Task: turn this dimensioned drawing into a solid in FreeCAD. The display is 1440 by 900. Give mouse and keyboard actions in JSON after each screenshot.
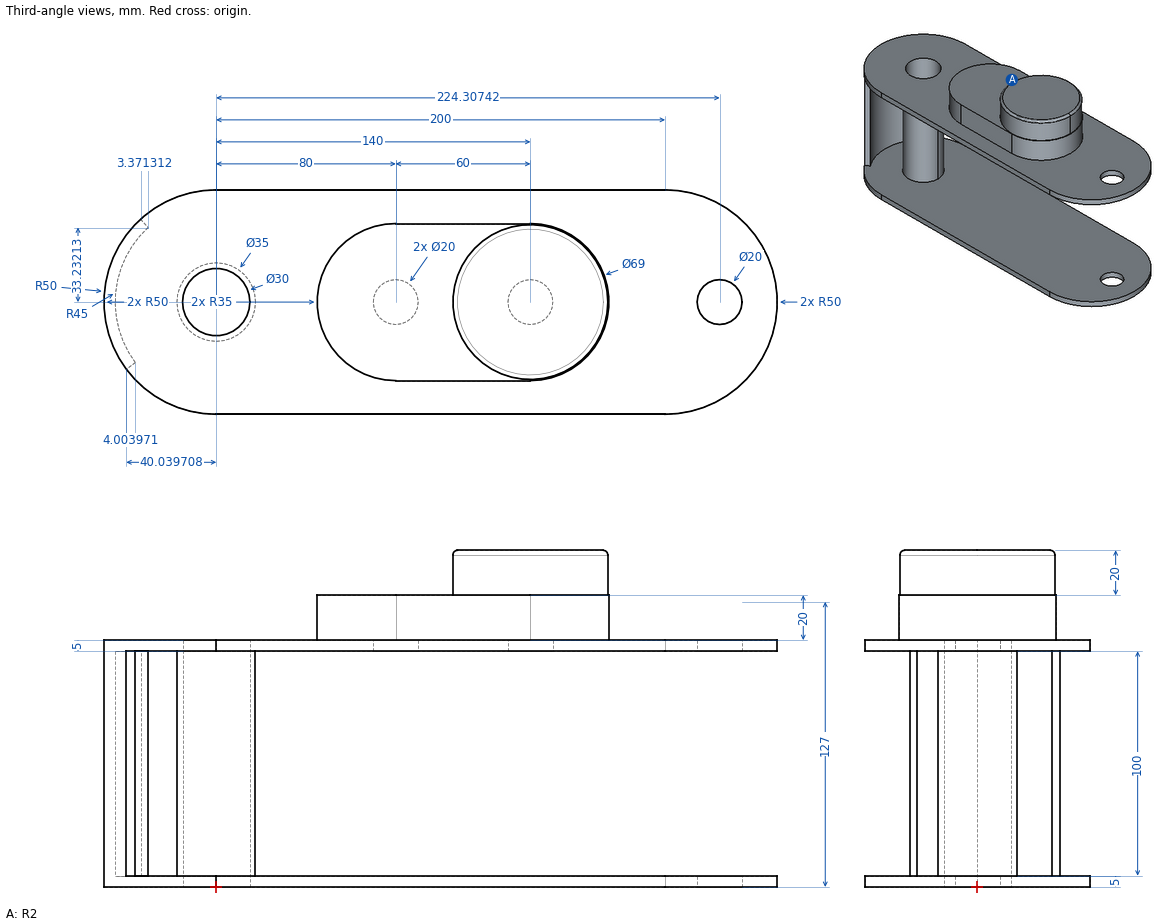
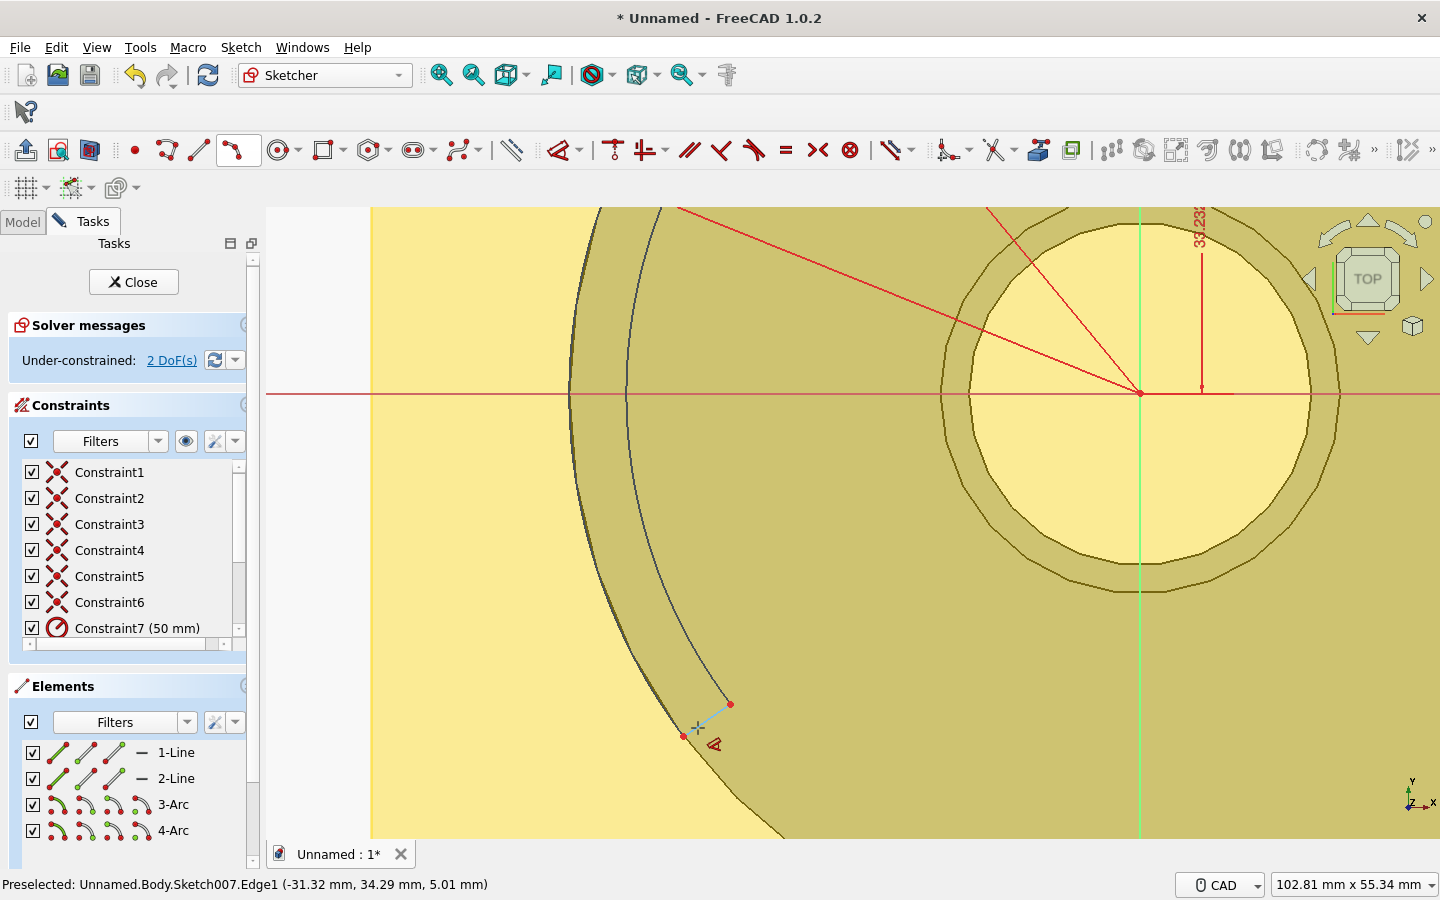
{"action": "left_click", "coordinate": [698, 727]}
{"action": "left_click", "coordinate": [707, 771]}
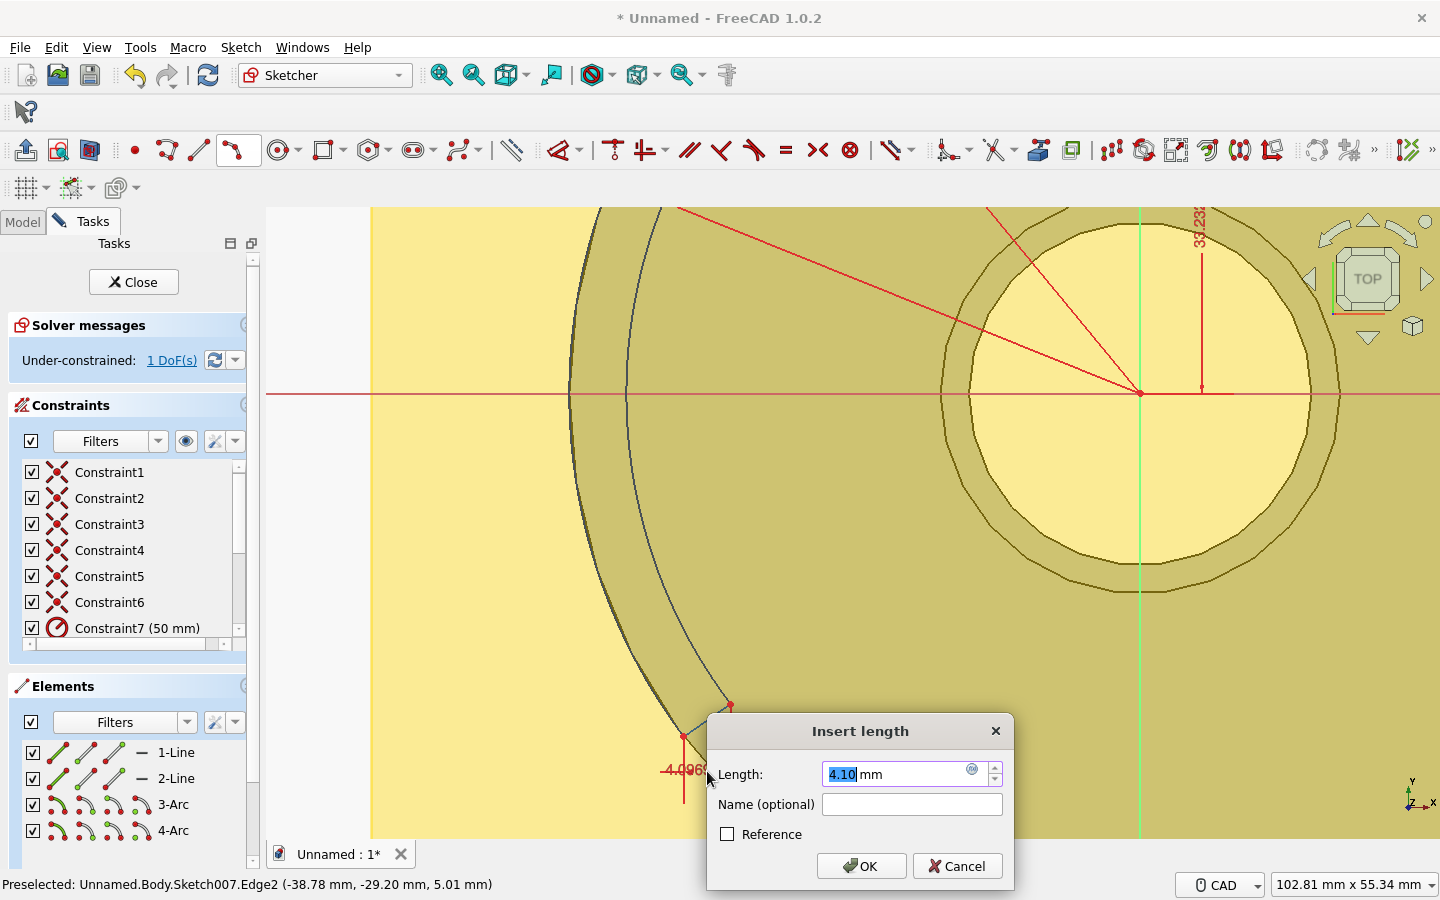
{"action": "type", "text": "4.003971"}
{"action": "key", "text": "Return"}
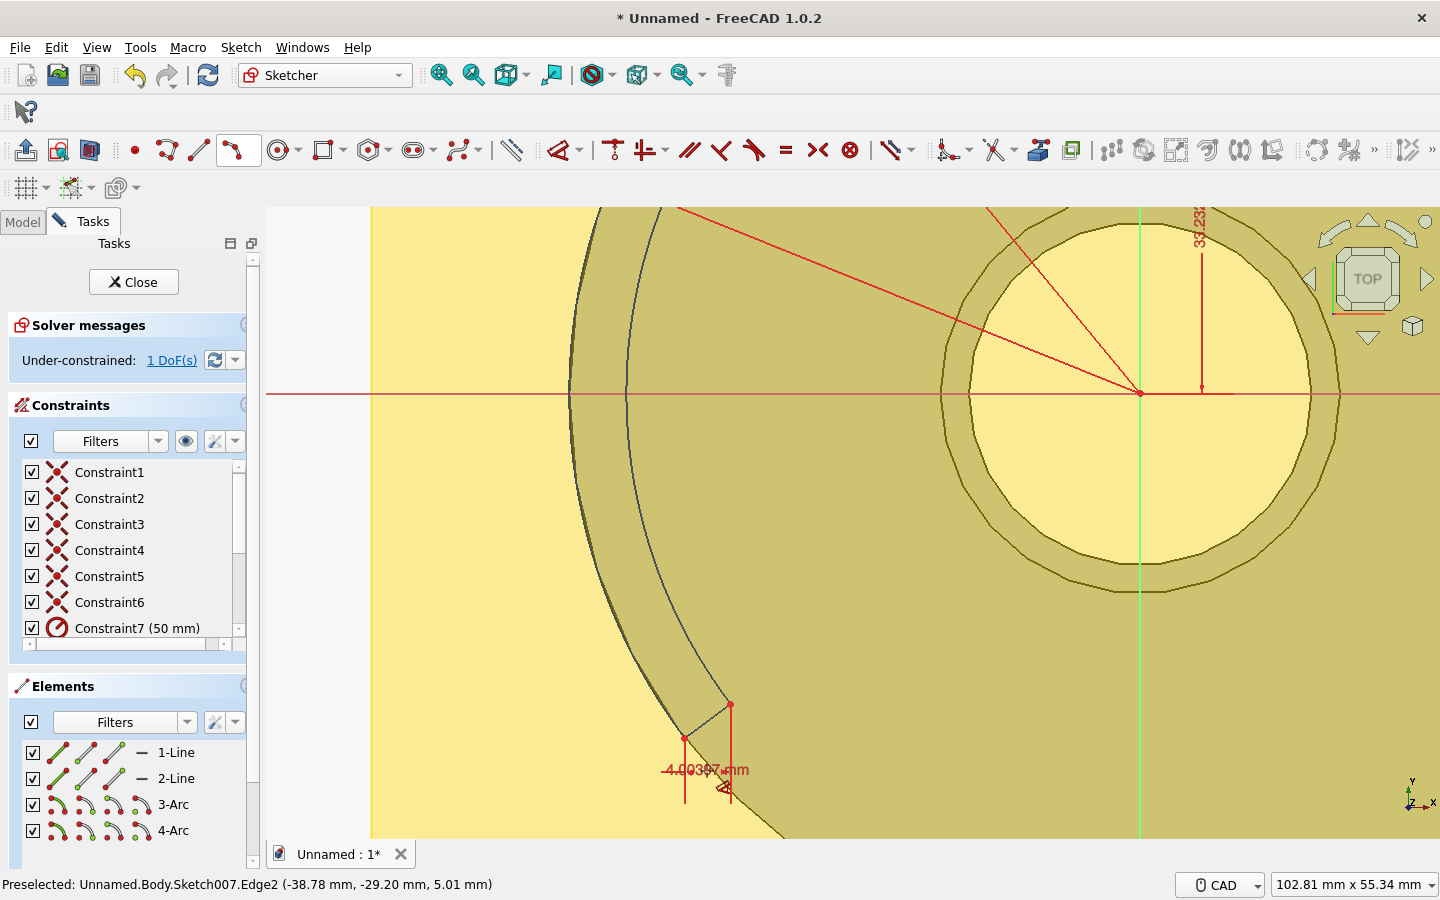
{"action": "left_click", "coordinate": [685, 738]}
{"action": "left_click", "coordinate": [913, 772]}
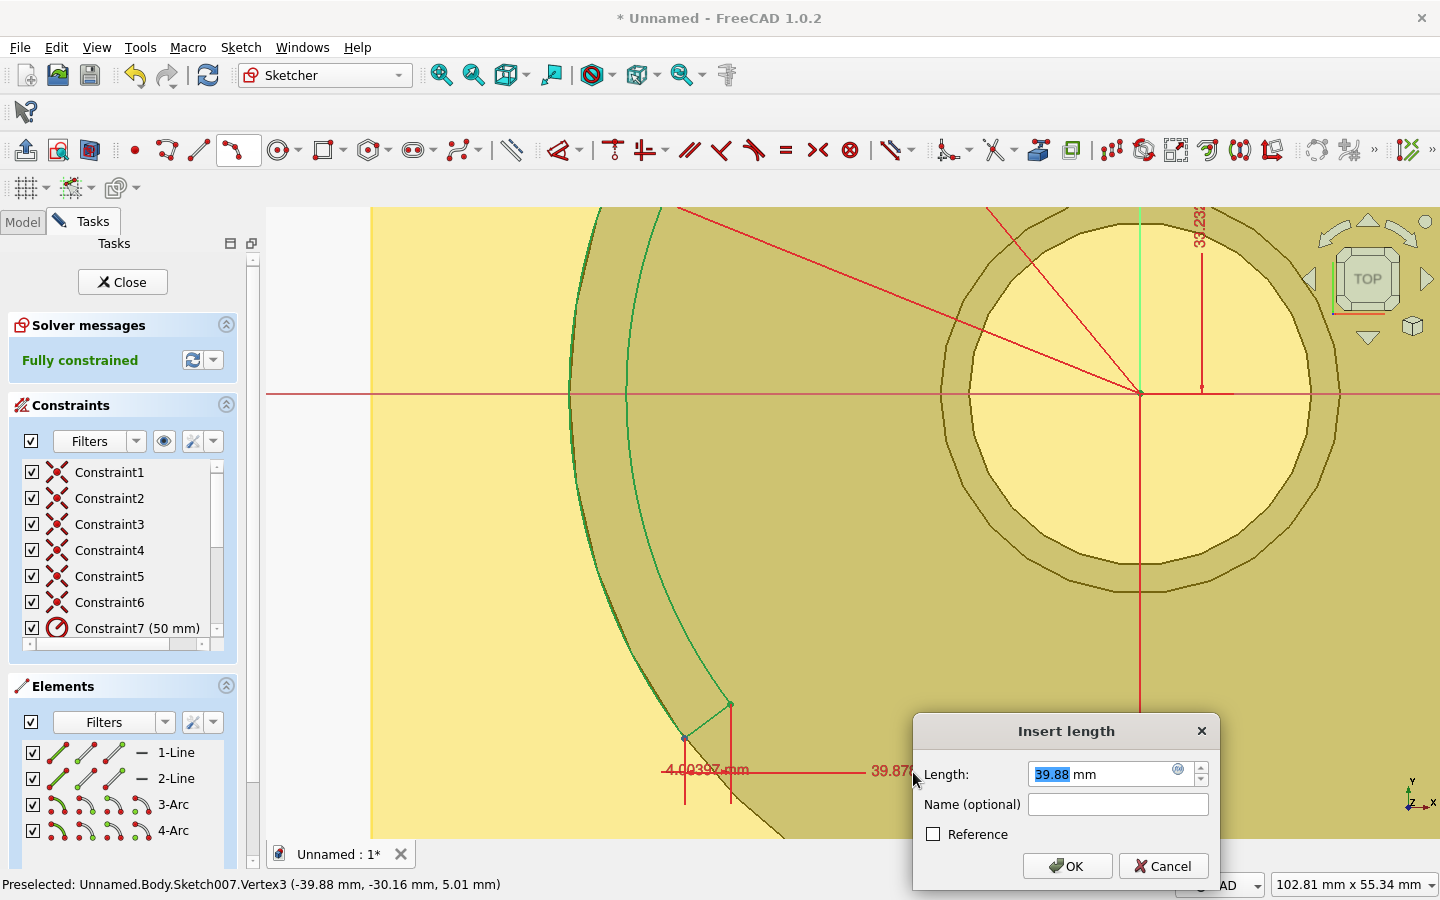
{"action": "type", "text": "40.039708"}
{"action": "key", "text": "Return"}
{"action": "key", "text": "Escape"}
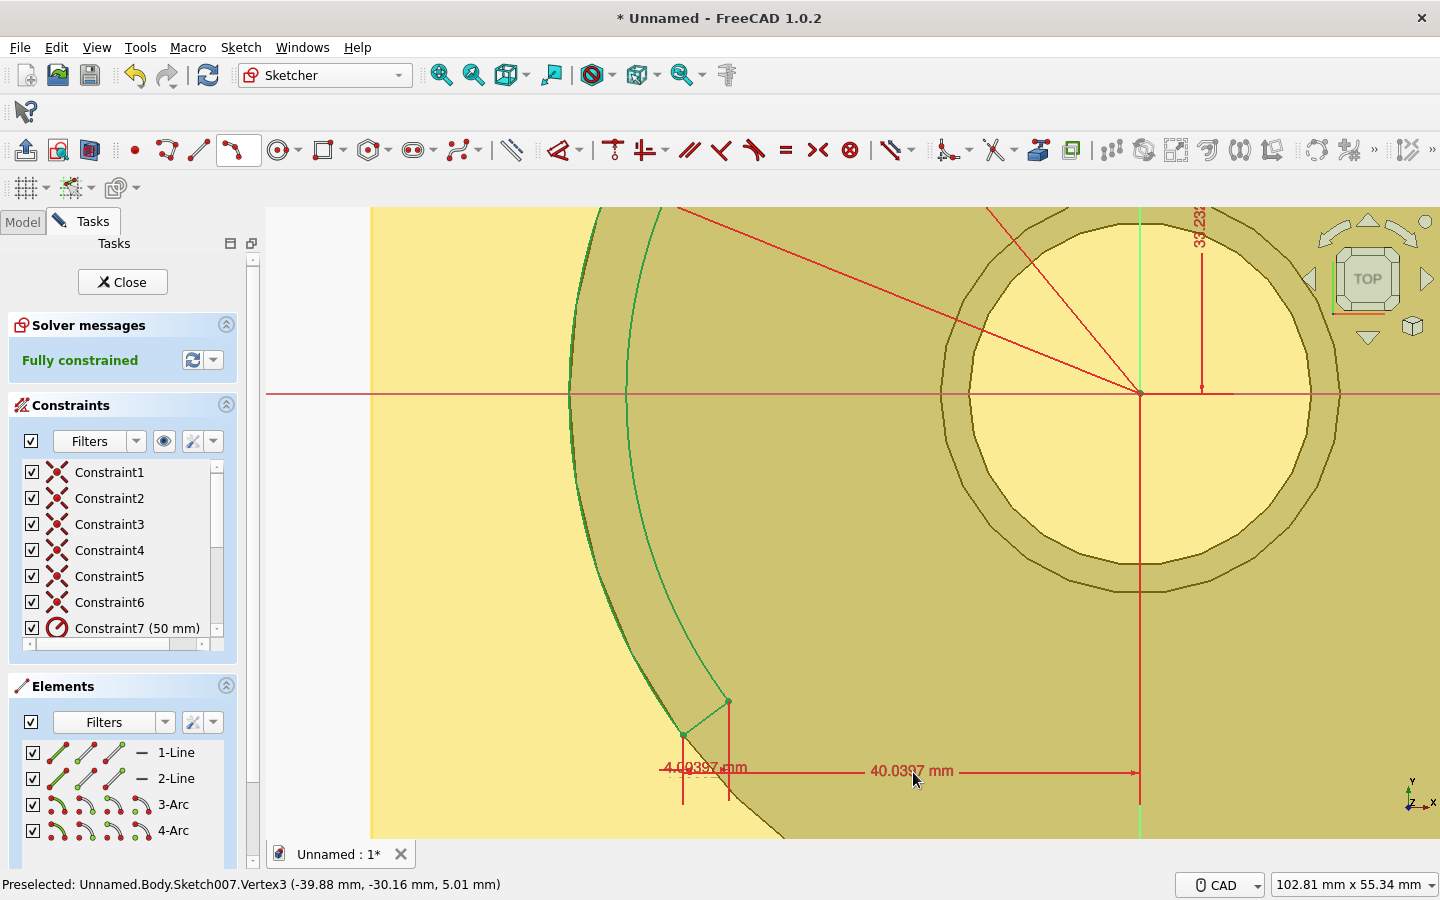
{"action": "left_click", "coordinate": [123, 282]}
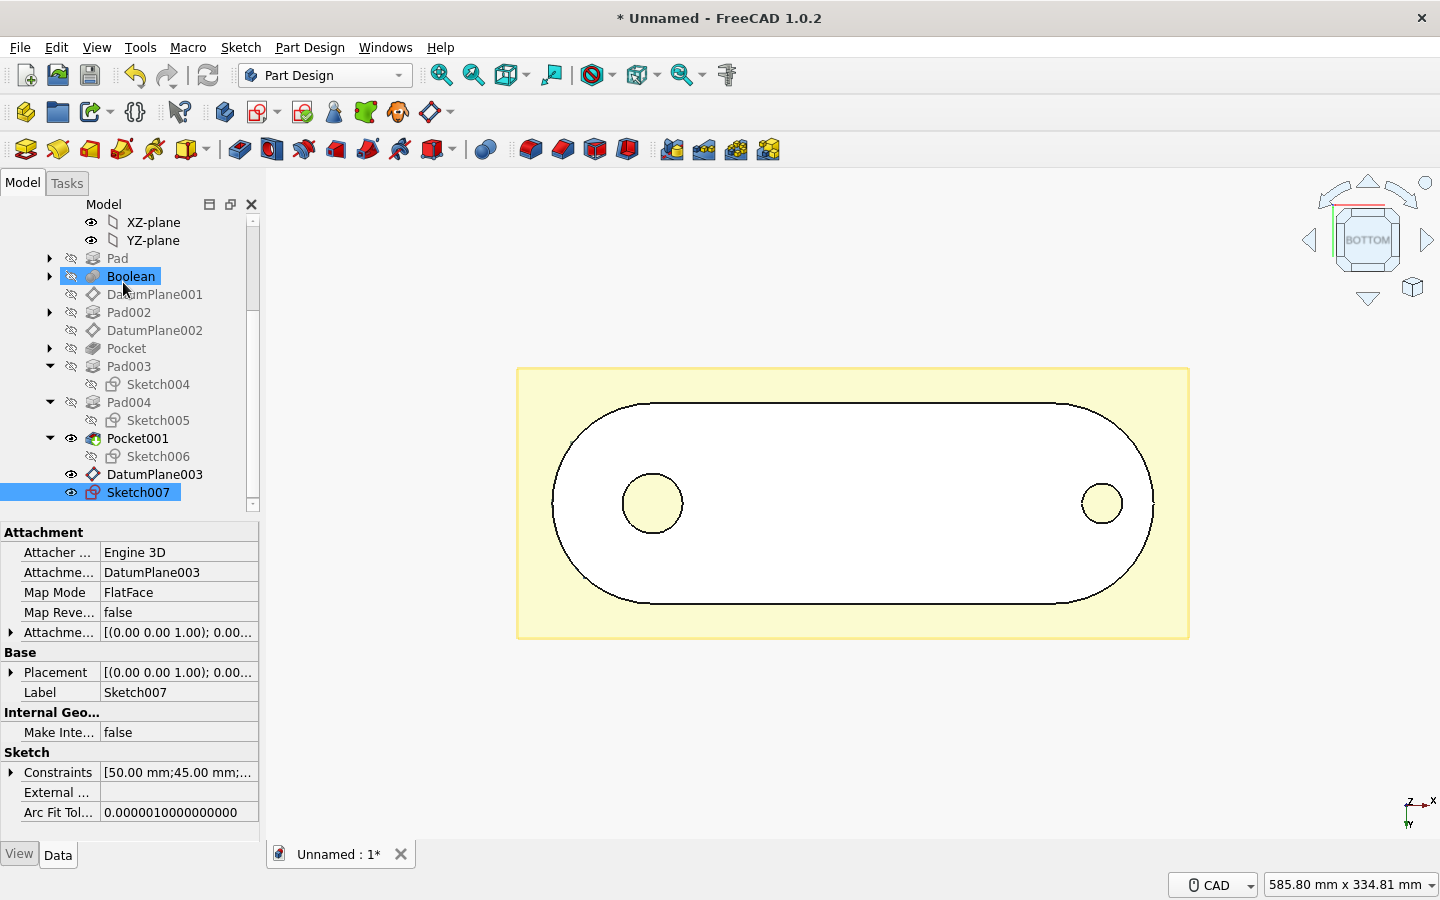
{"action": "left_click", "coordinate": [26, 150]}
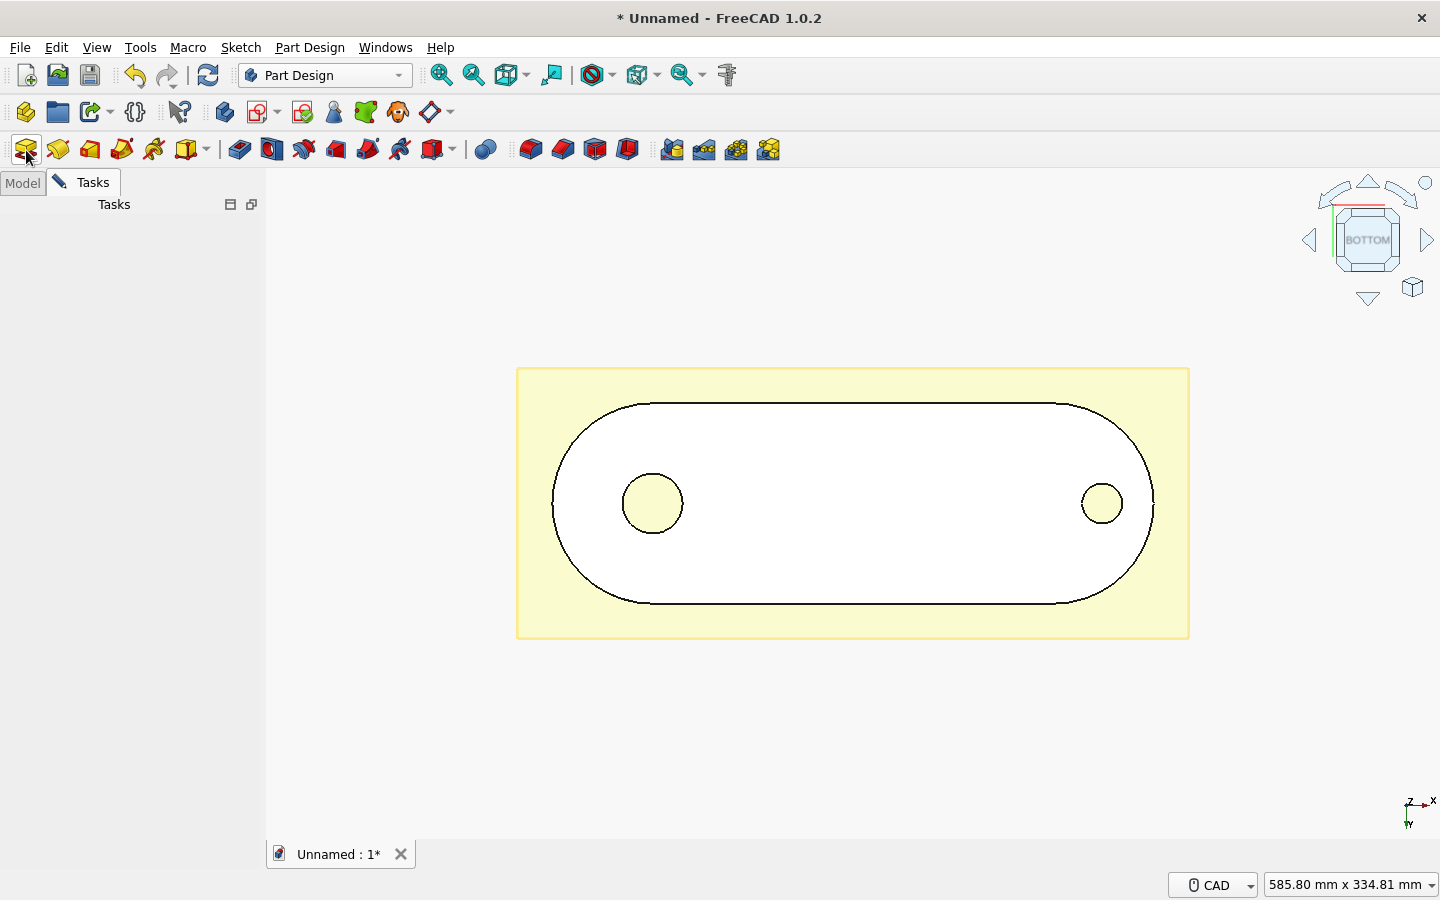
{"action": "left_click", "coordinate": [212, 324]}